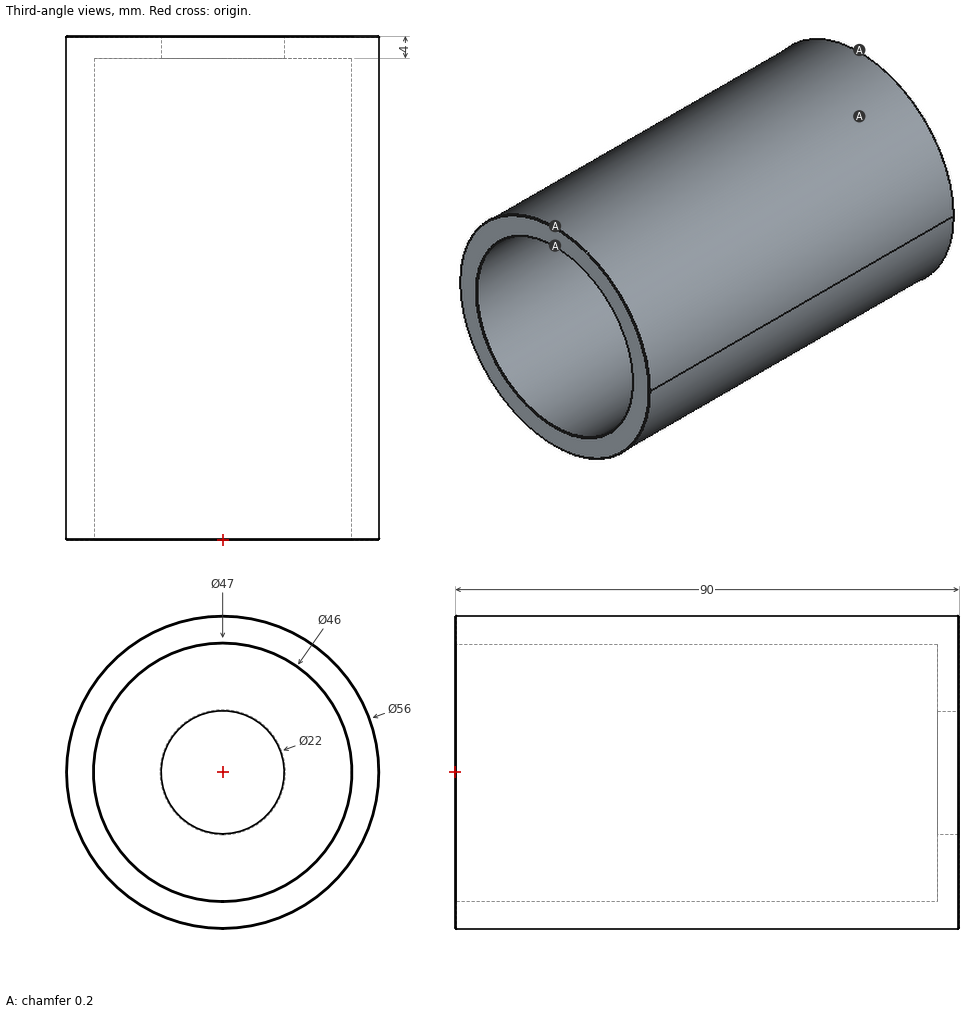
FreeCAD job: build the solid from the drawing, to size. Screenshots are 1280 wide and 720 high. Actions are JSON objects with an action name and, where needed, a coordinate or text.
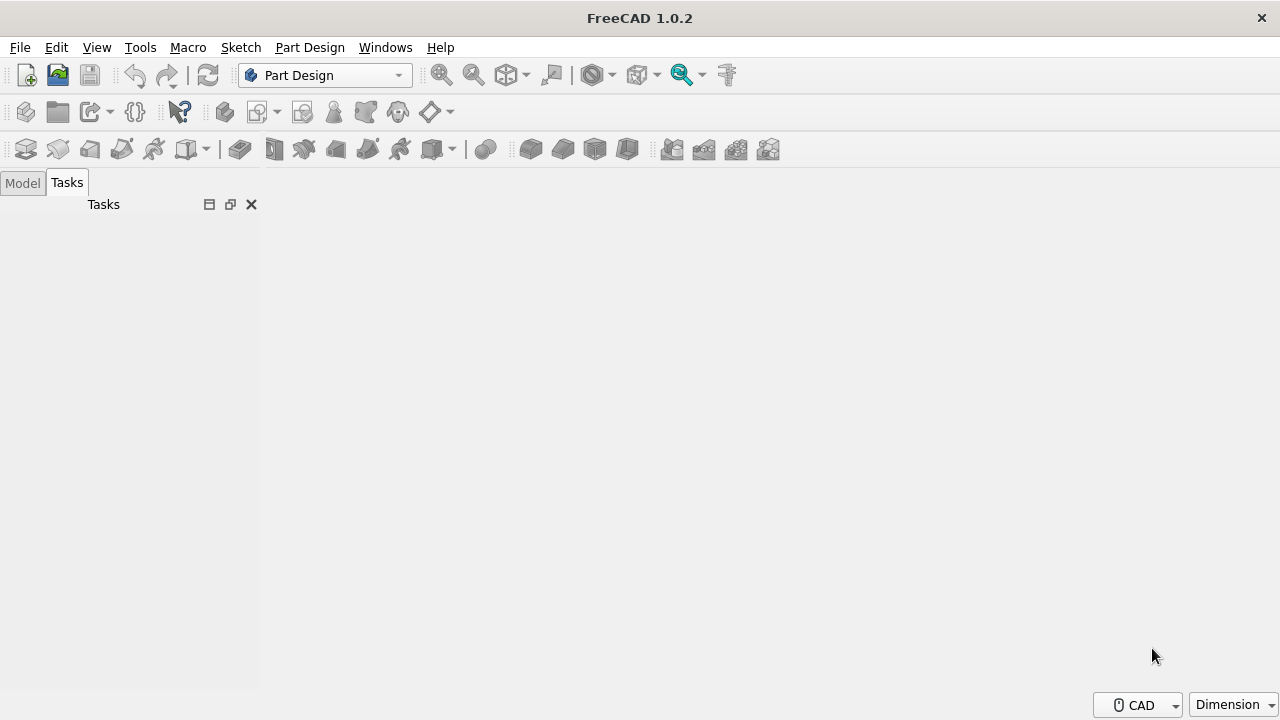
{"action": "left_click", "coordinate": [616, 76]}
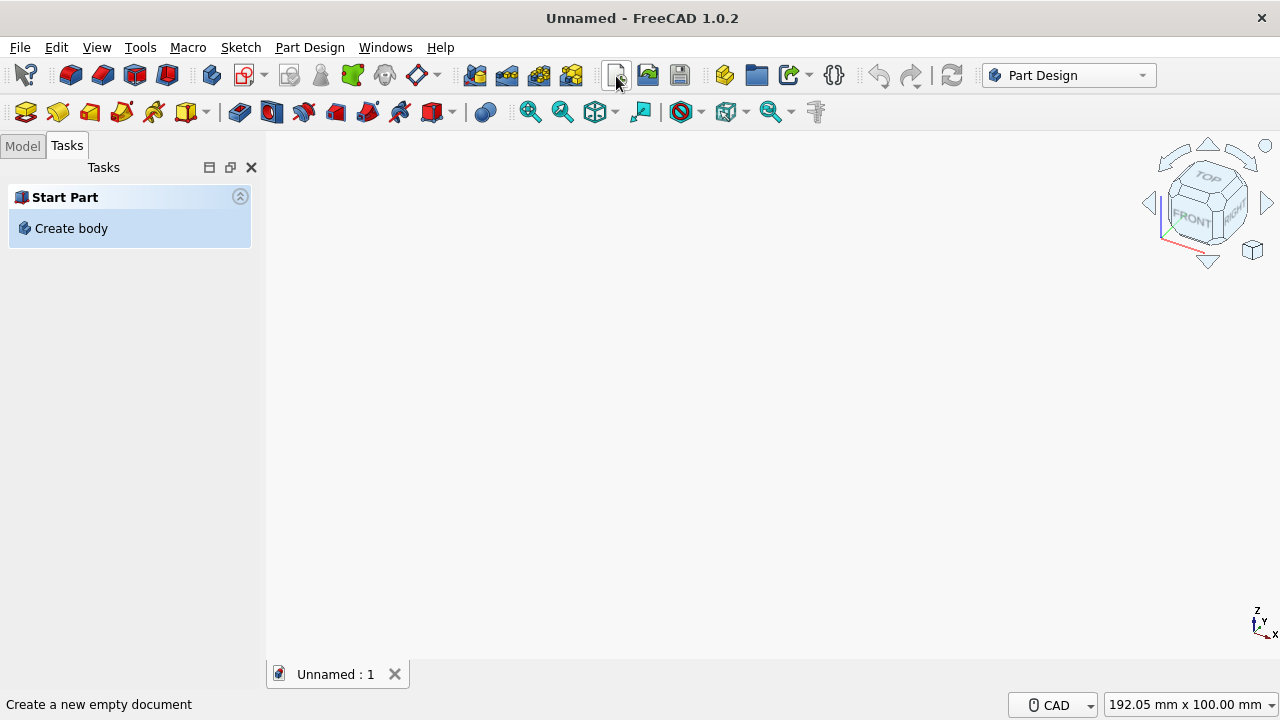
{"action": "left_click", "coordinate": [244, 76]}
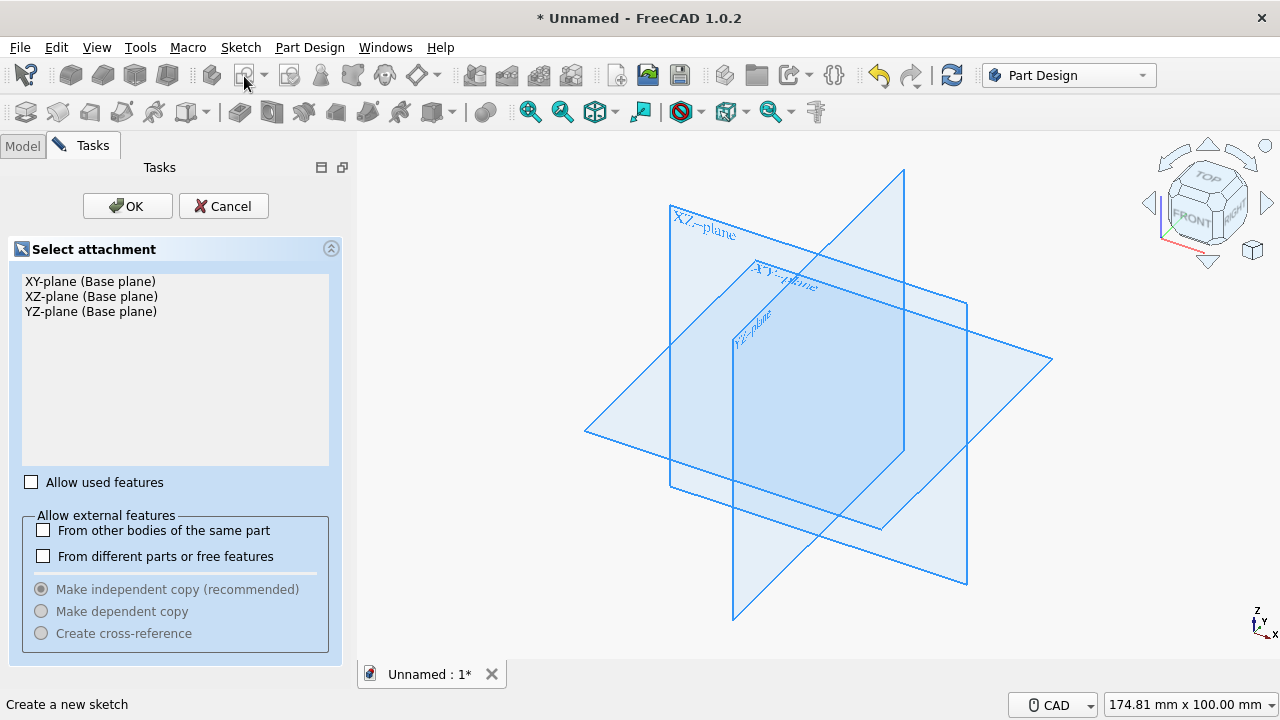
{"action": "left_click", "coordinate": [82, 296]}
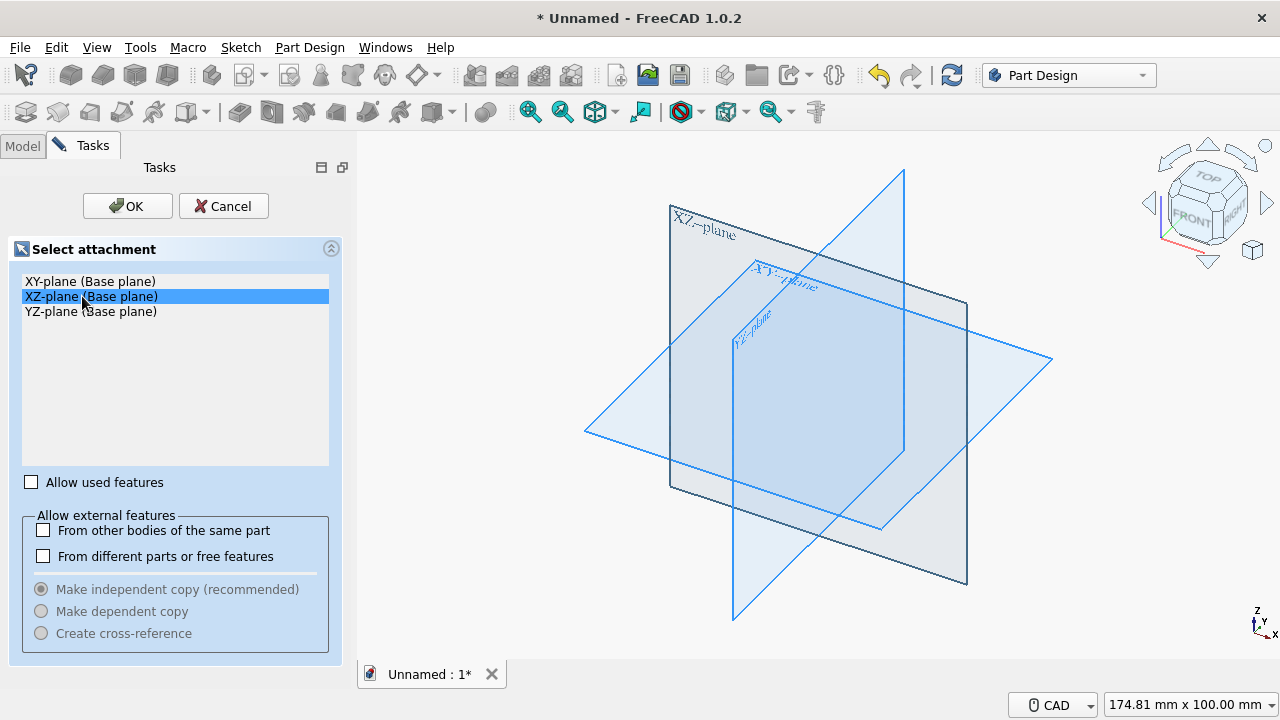
{"action": "left_click", "coordinate": [128, 206]}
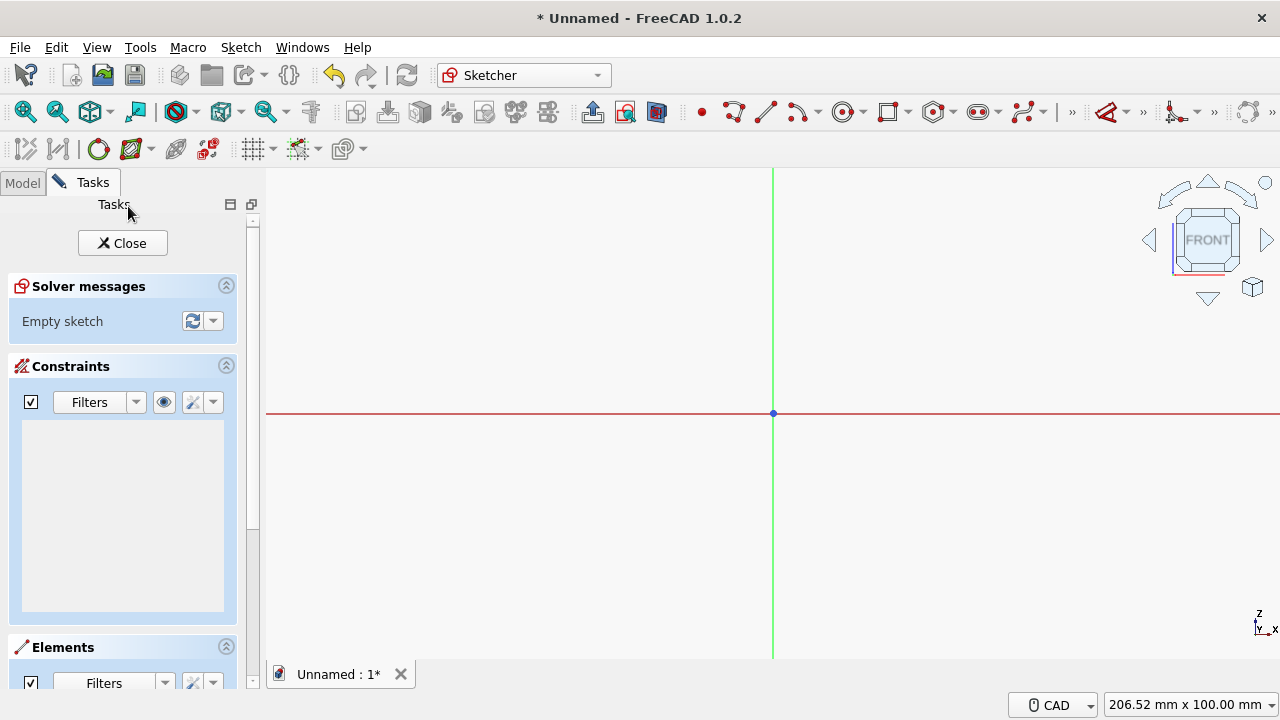
{"action": "left_click", "coordinate": [844, 112]}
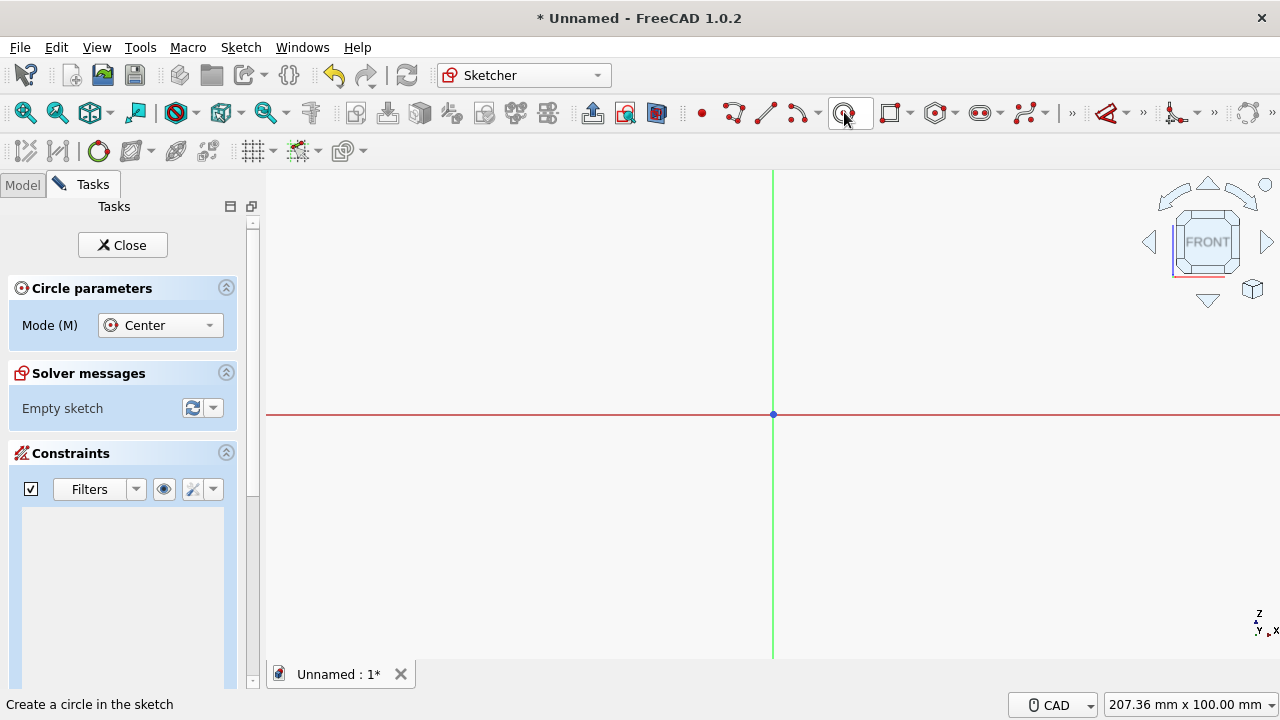
{"action": "left_click", "coordinate": [773, 414]}
{"action": "left_click", "coordinate": [870, 318]}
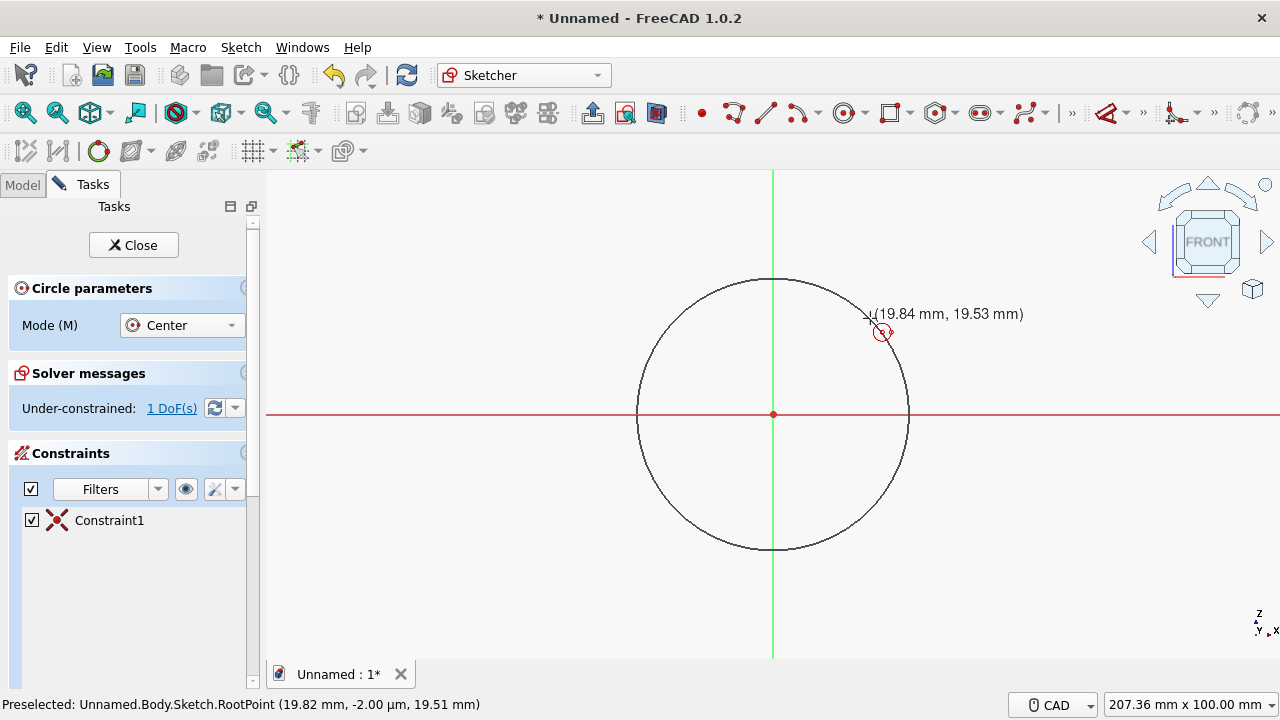
{"action": "left_click", "coordinate": [773, 414]}
{"action": "left_click", "coordinate": [853, 335]}
{"action": "key", "text": "Escape"}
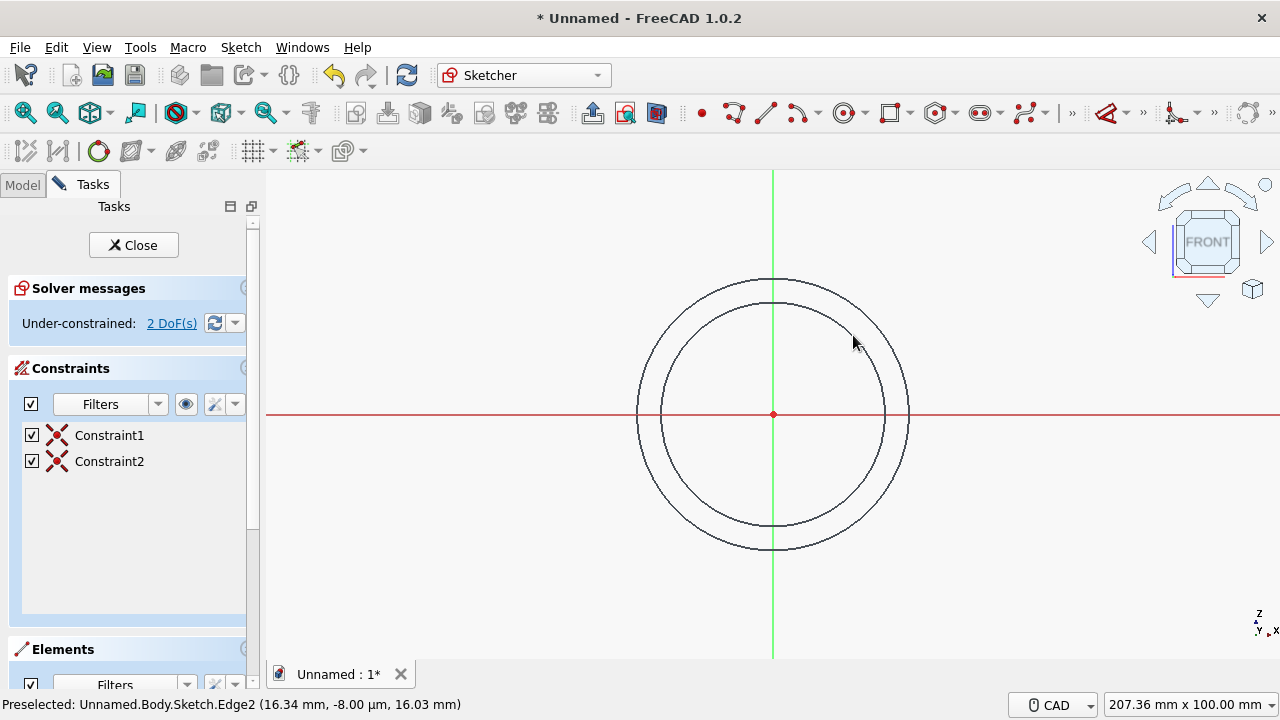
{"action": "left_click", "coordinate": [1106, 114]}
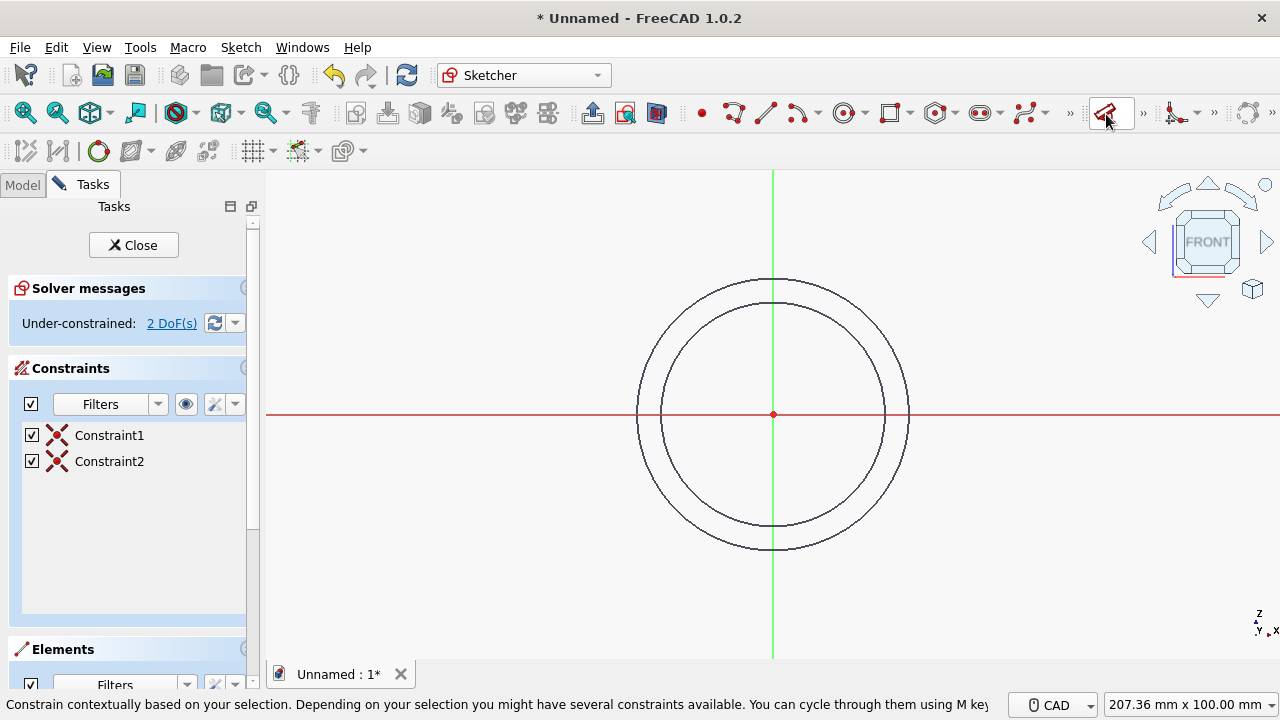
{"action": "left_click", "coordinate": [869, 318]}
{"action": "left_click", "coordinate": [892, 295]}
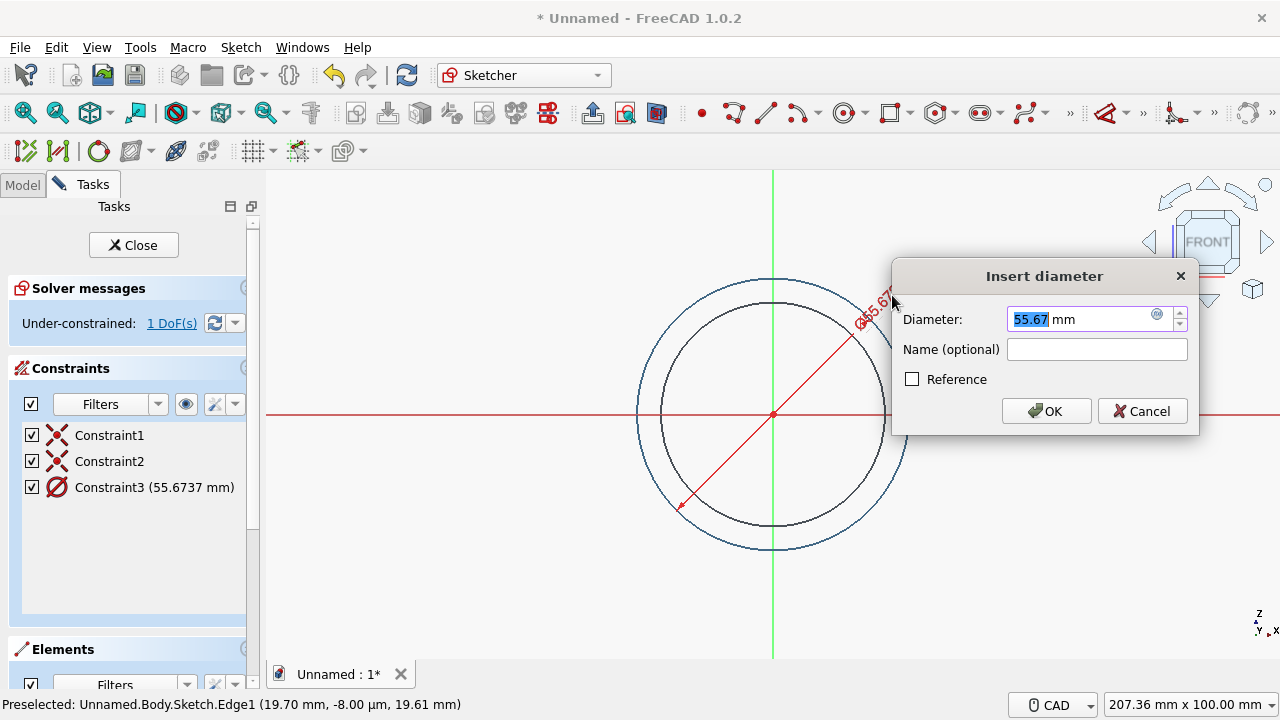
{"action": "type", "text": "56"}
{"action": "key", "text": "Return"}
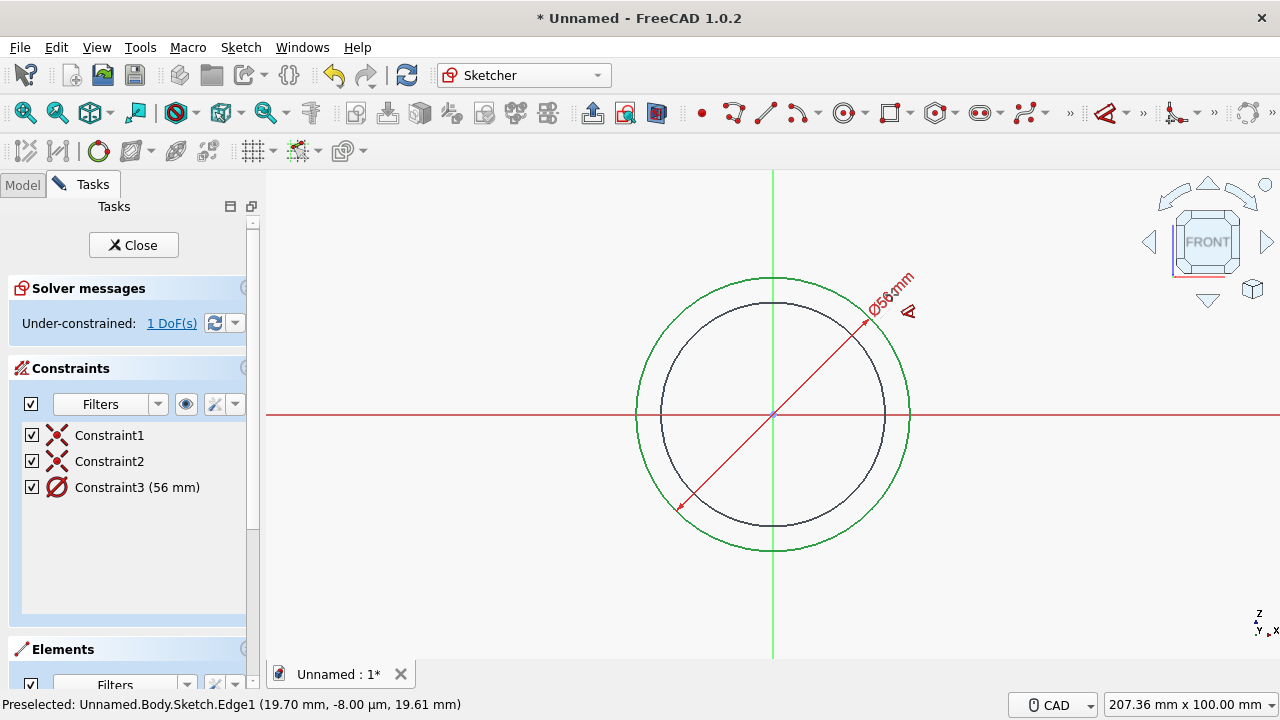
{"action": "left_click", "coordinate": [852, 335]}
{"action": "left_click", "coordinate": [933, 367]}